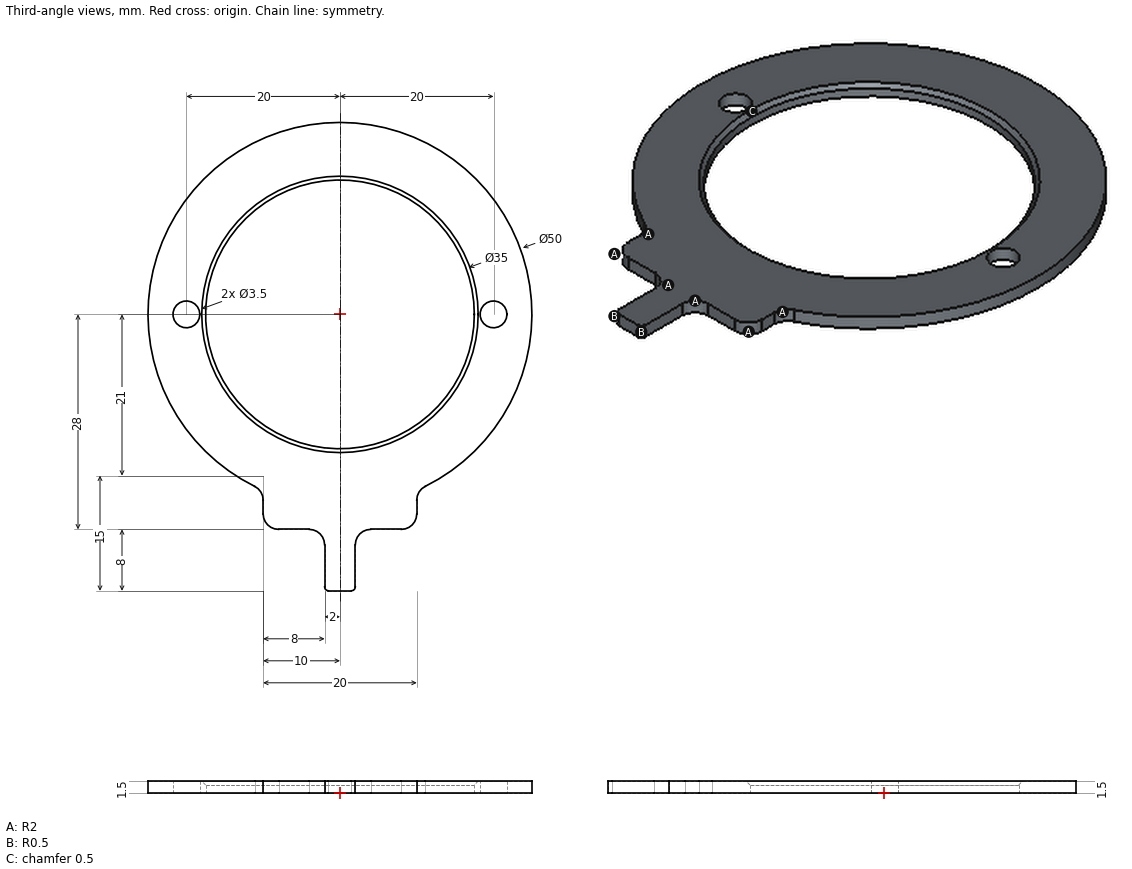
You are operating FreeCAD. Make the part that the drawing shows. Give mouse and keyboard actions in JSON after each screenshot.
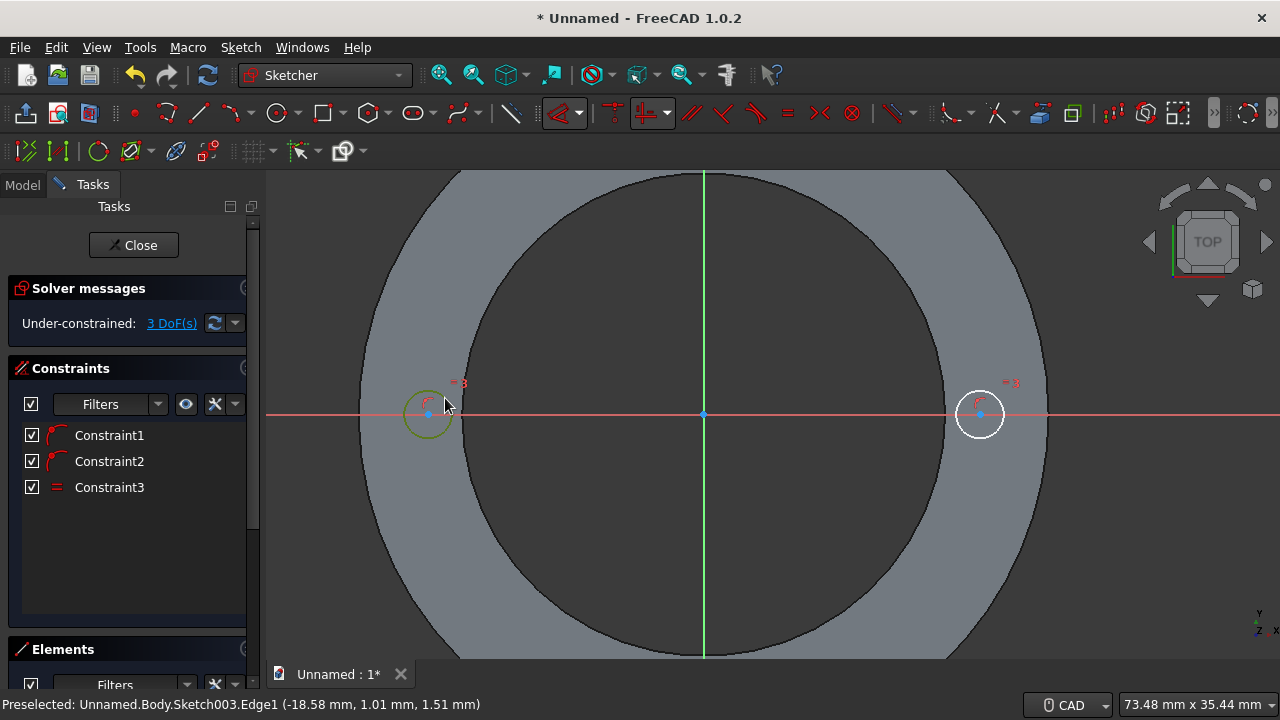
{"action": "left_click", "coordinate": [582, 114]}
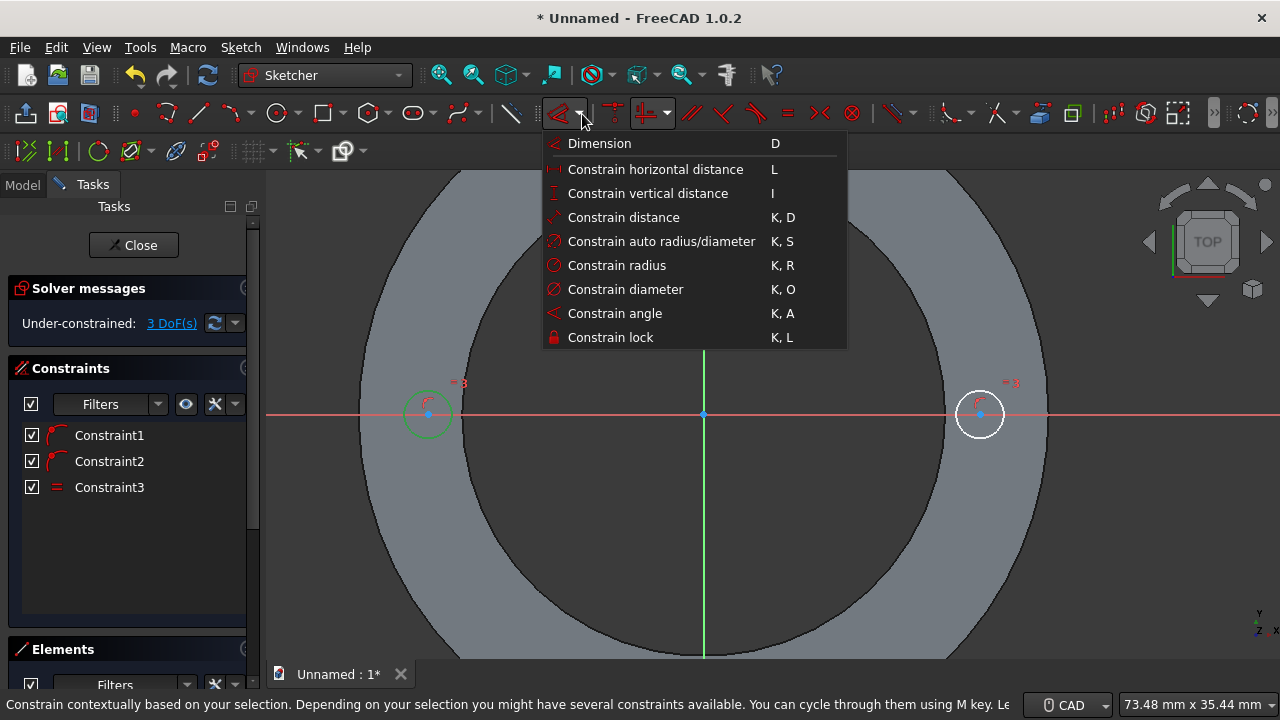
{"action": "left_click", "coordinate": [695, 289]}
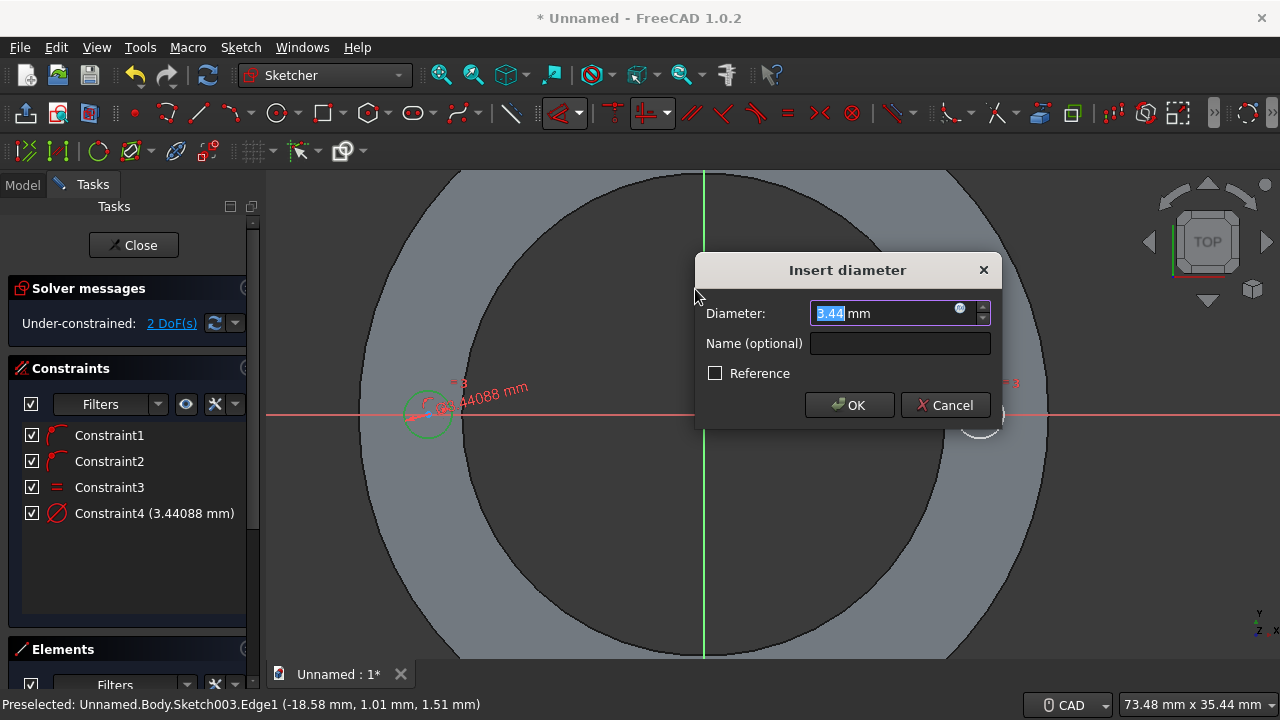
{"action": "type", "text": "3.5"}
{"action": "key", "text": "Return"}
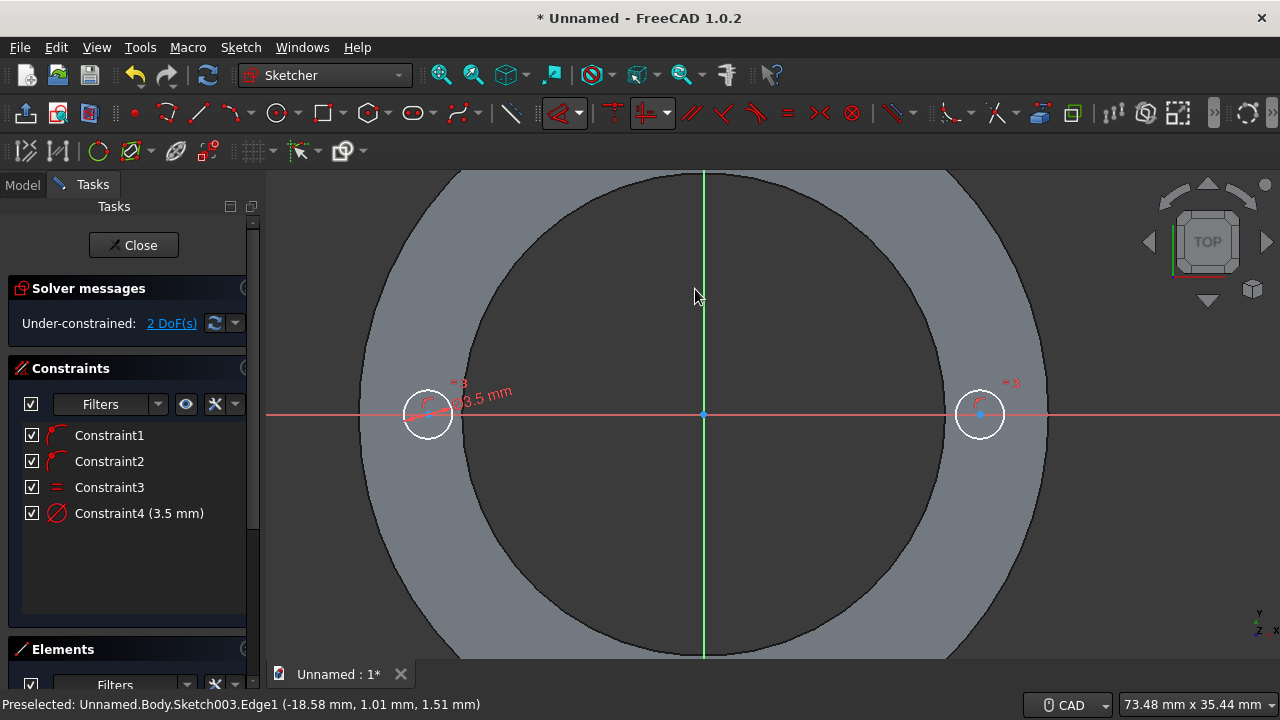
{"action": "left_click", "coordinate": [428, 415]}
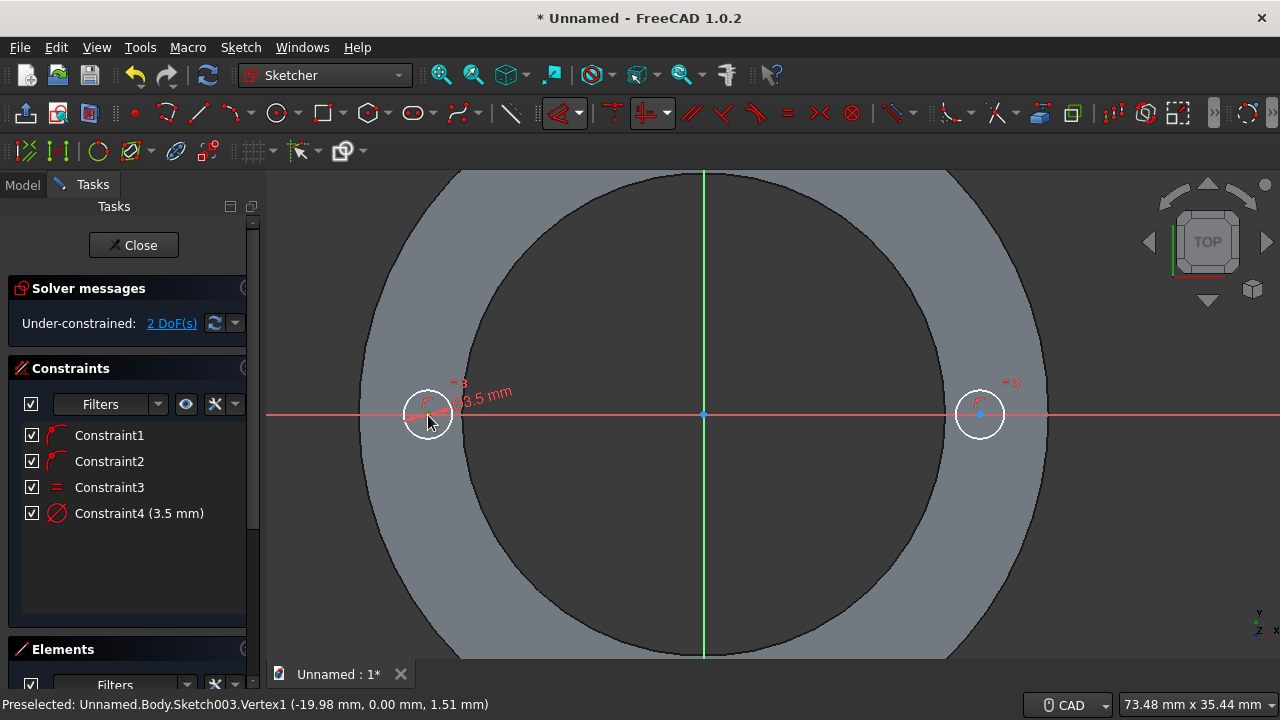
{"action": "key", "text": "l"}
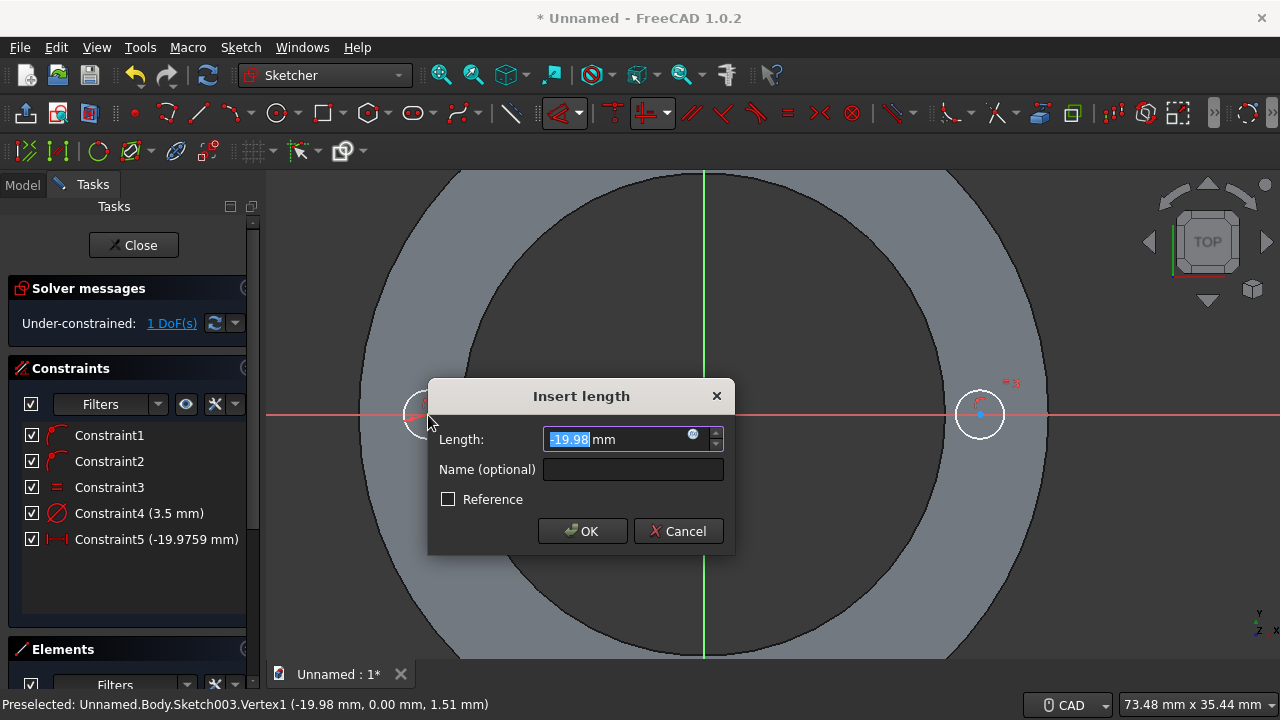
{"action": "type", "text": "-20"}
{"action": "key", "text": "Return"}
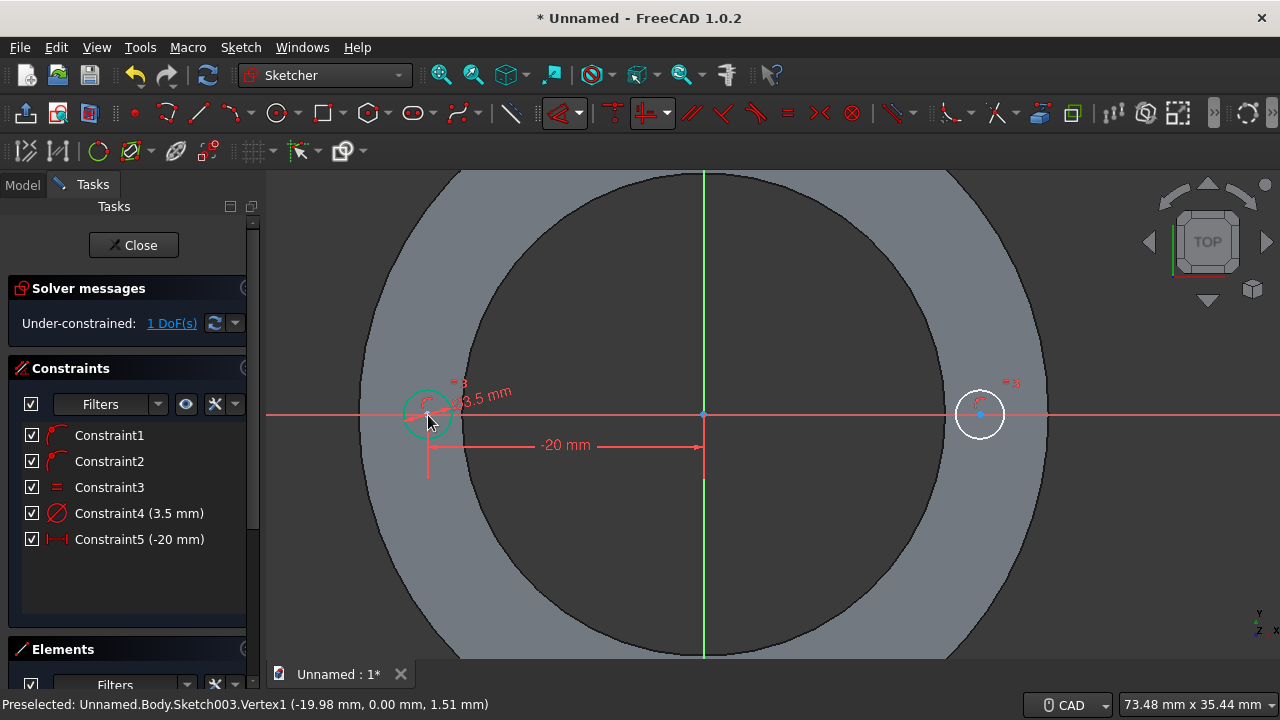
{"action": "left_click", "coordinate": [980, 415]}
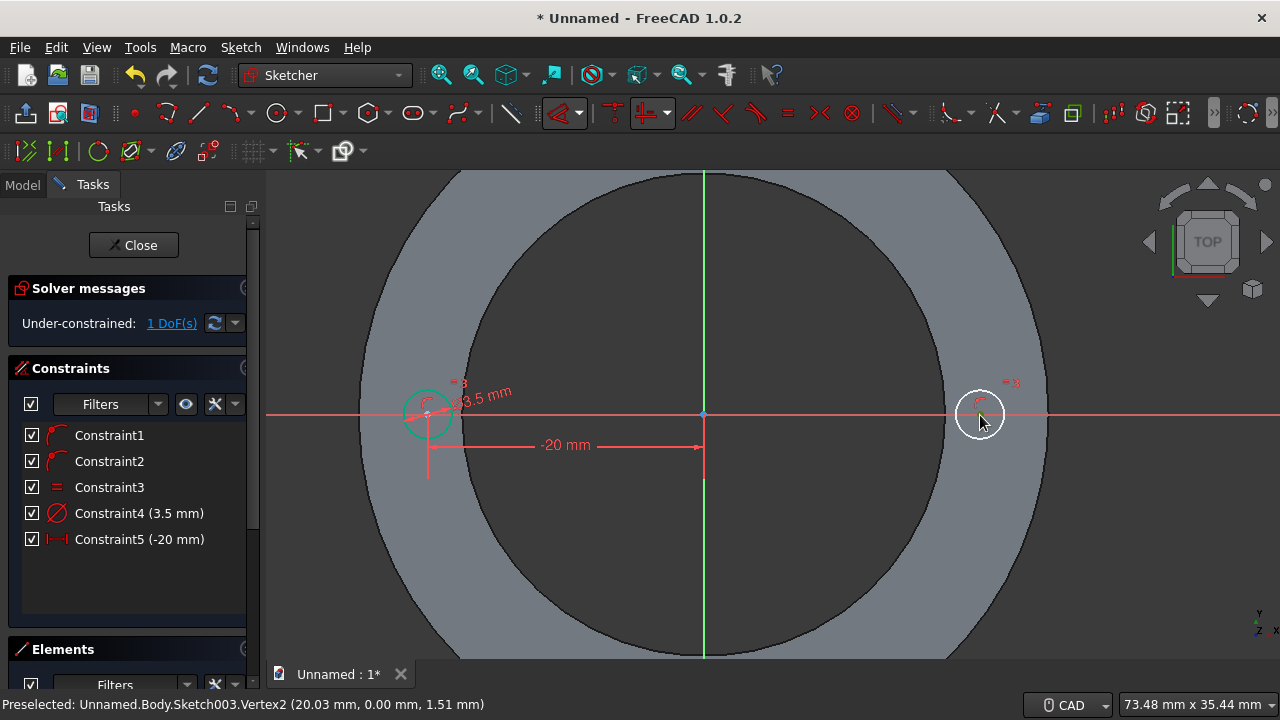
{"action": "left_click", "coordinate": [582, 114]}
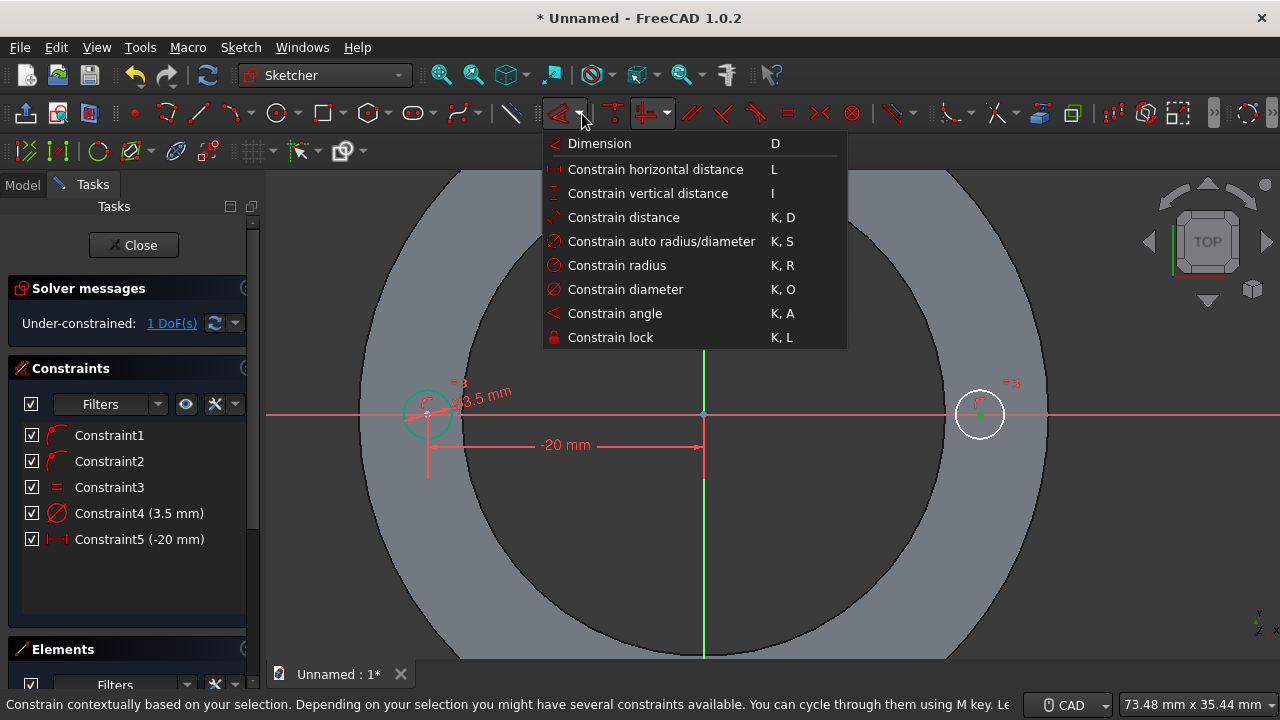
{"action": "left_click", "coordinate": [695, 169]}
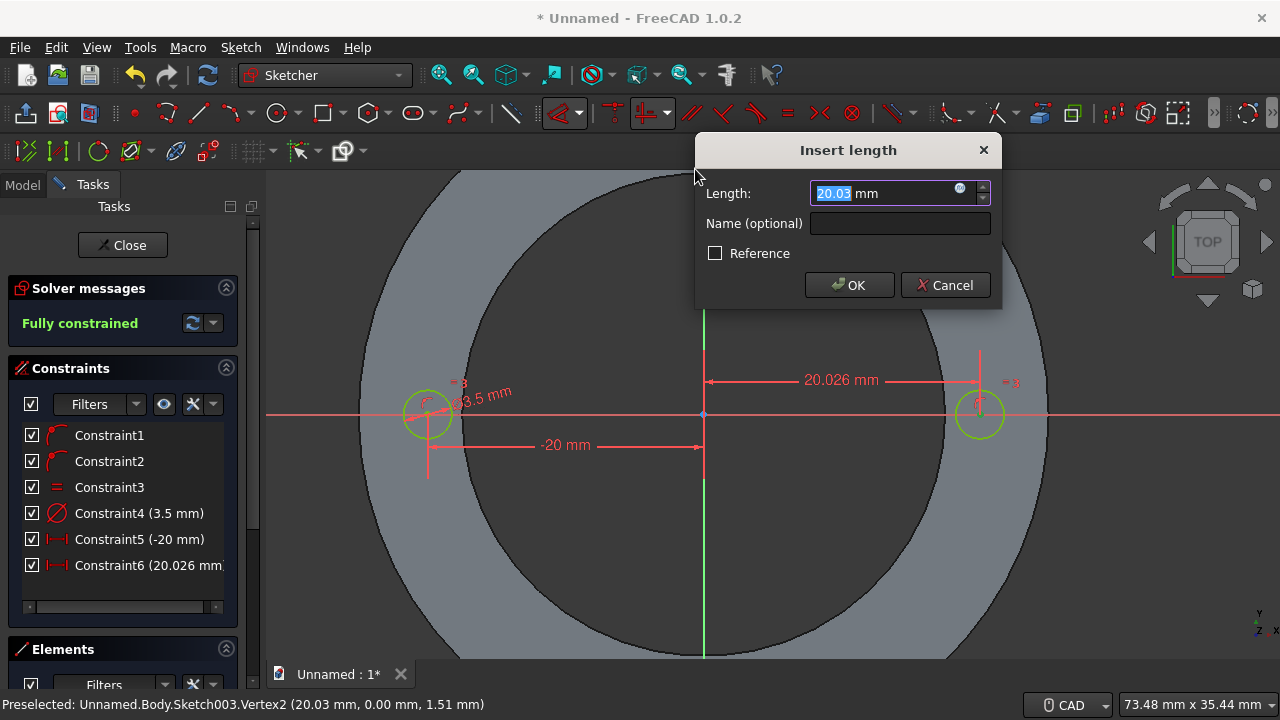
{"action": "type", "text": "20"}
{"action": "key", "text": "Return"}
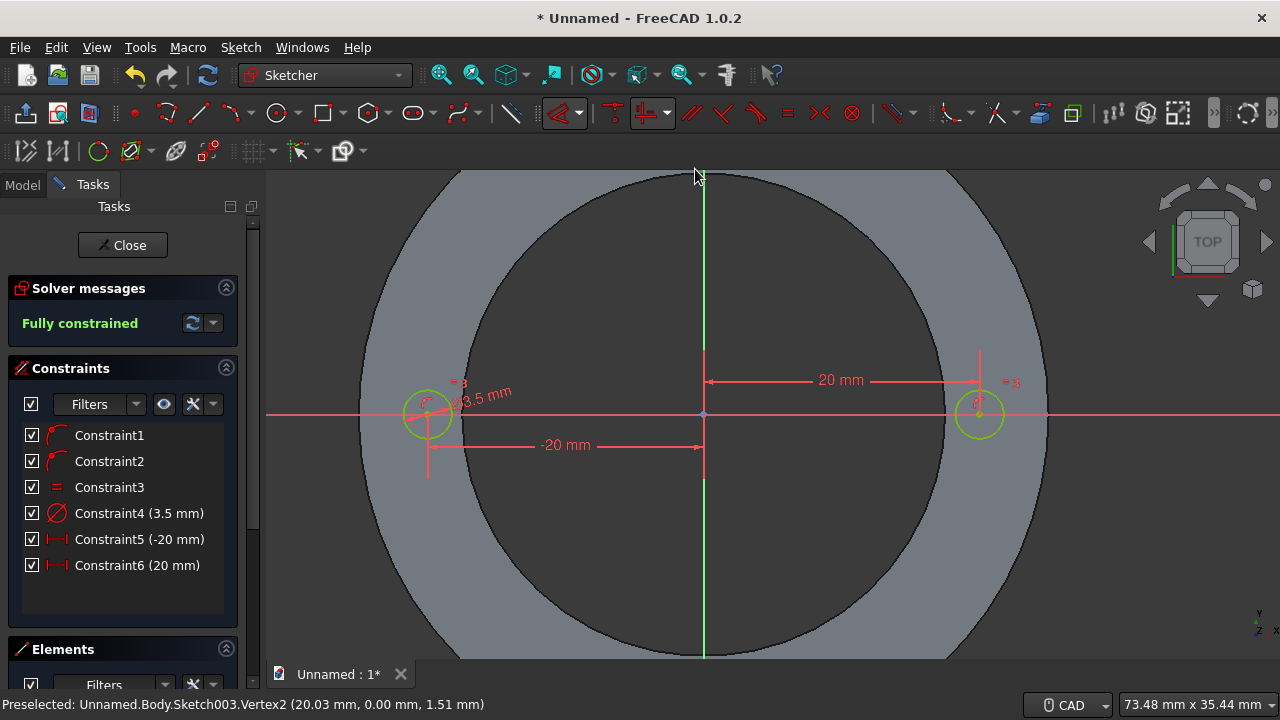
{"action": "left_click", "coordinate": [123, 245]}